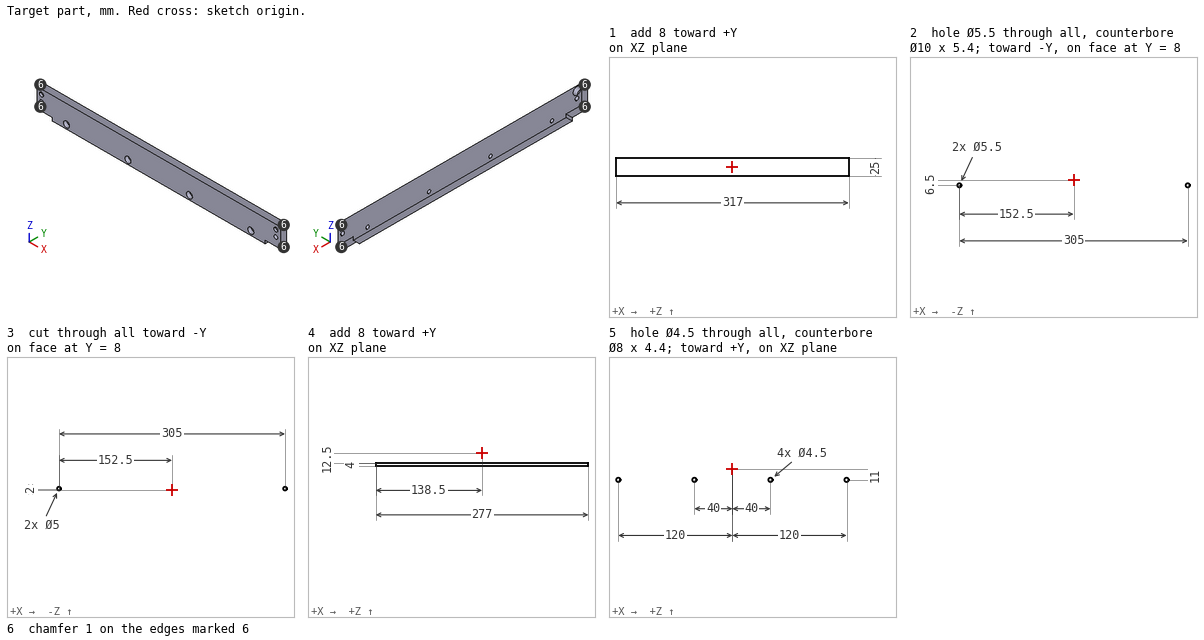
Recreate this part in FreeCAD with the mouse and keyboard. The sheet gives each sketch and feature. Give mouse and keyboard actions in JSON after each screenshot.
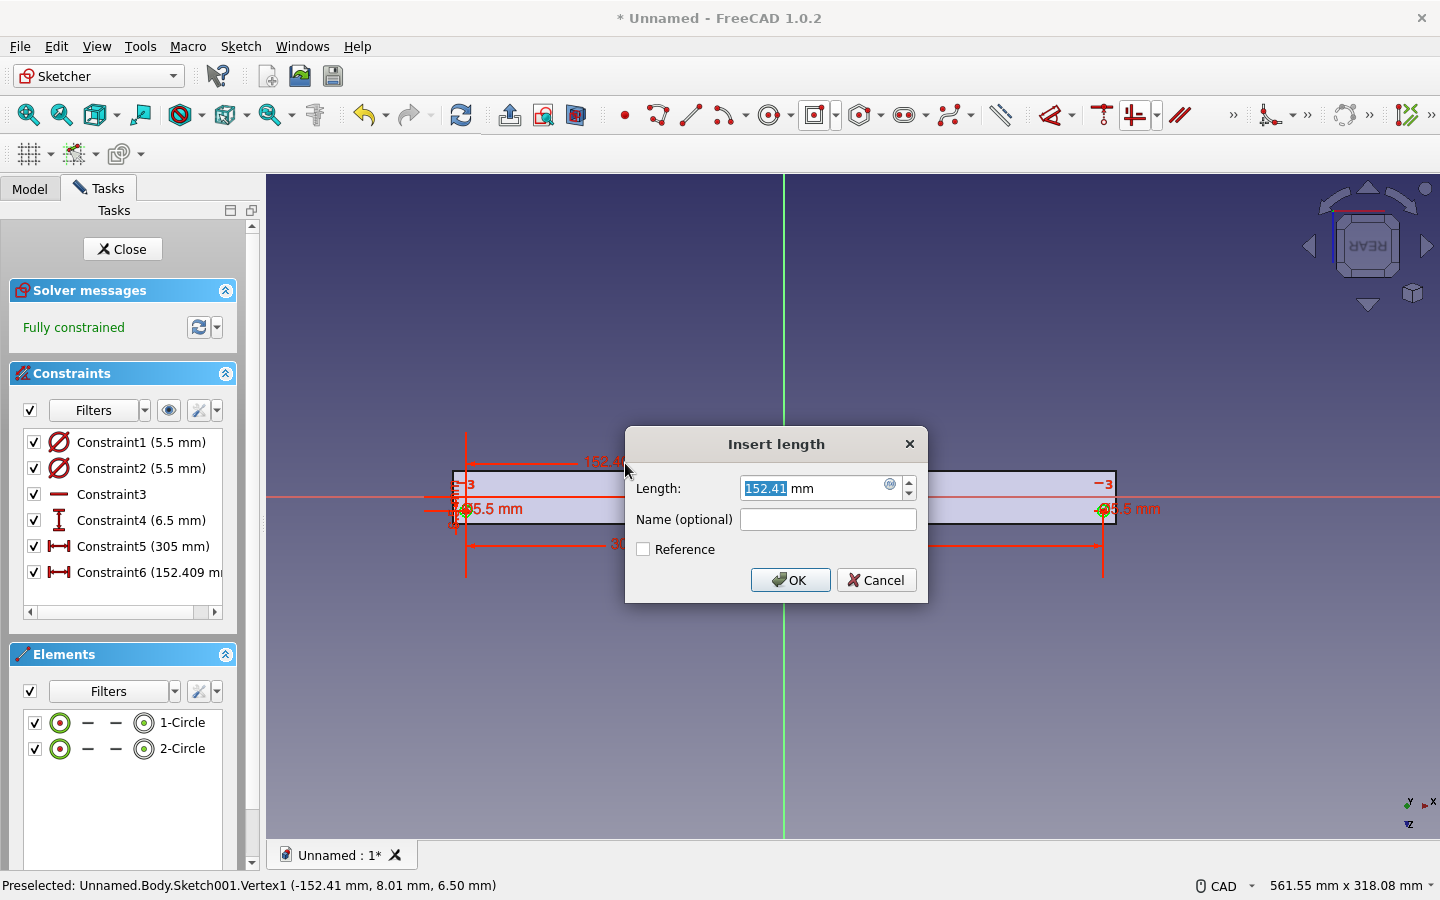
{"action": "type", "text": "152.5"}
{"action": "key", "text": "Return"}
{"action": "key", "text": "Escape"}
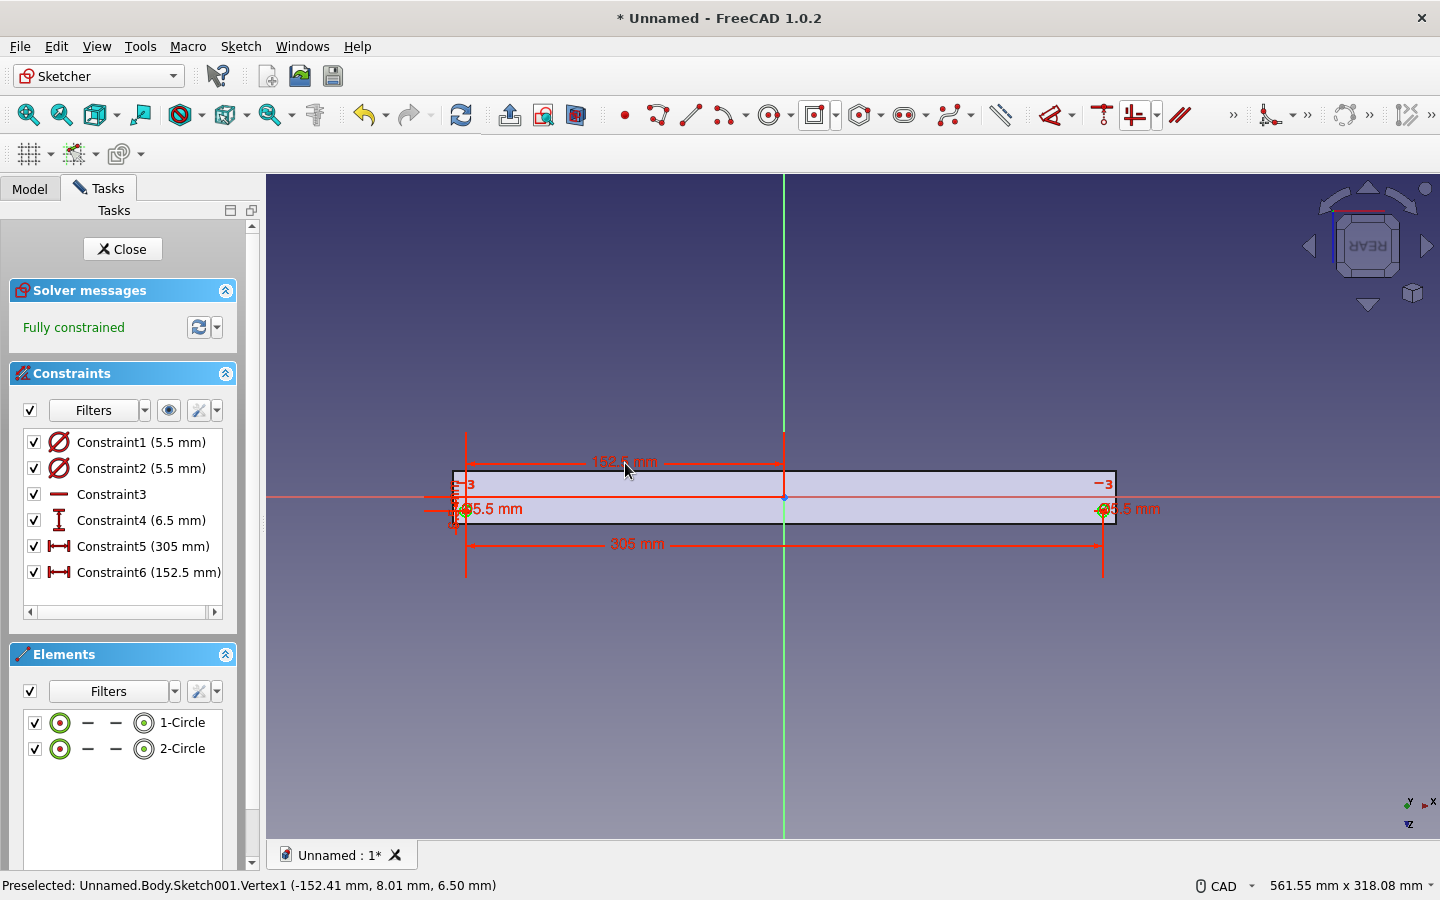
{"action": "left_click", "coordinate": [123, 249]}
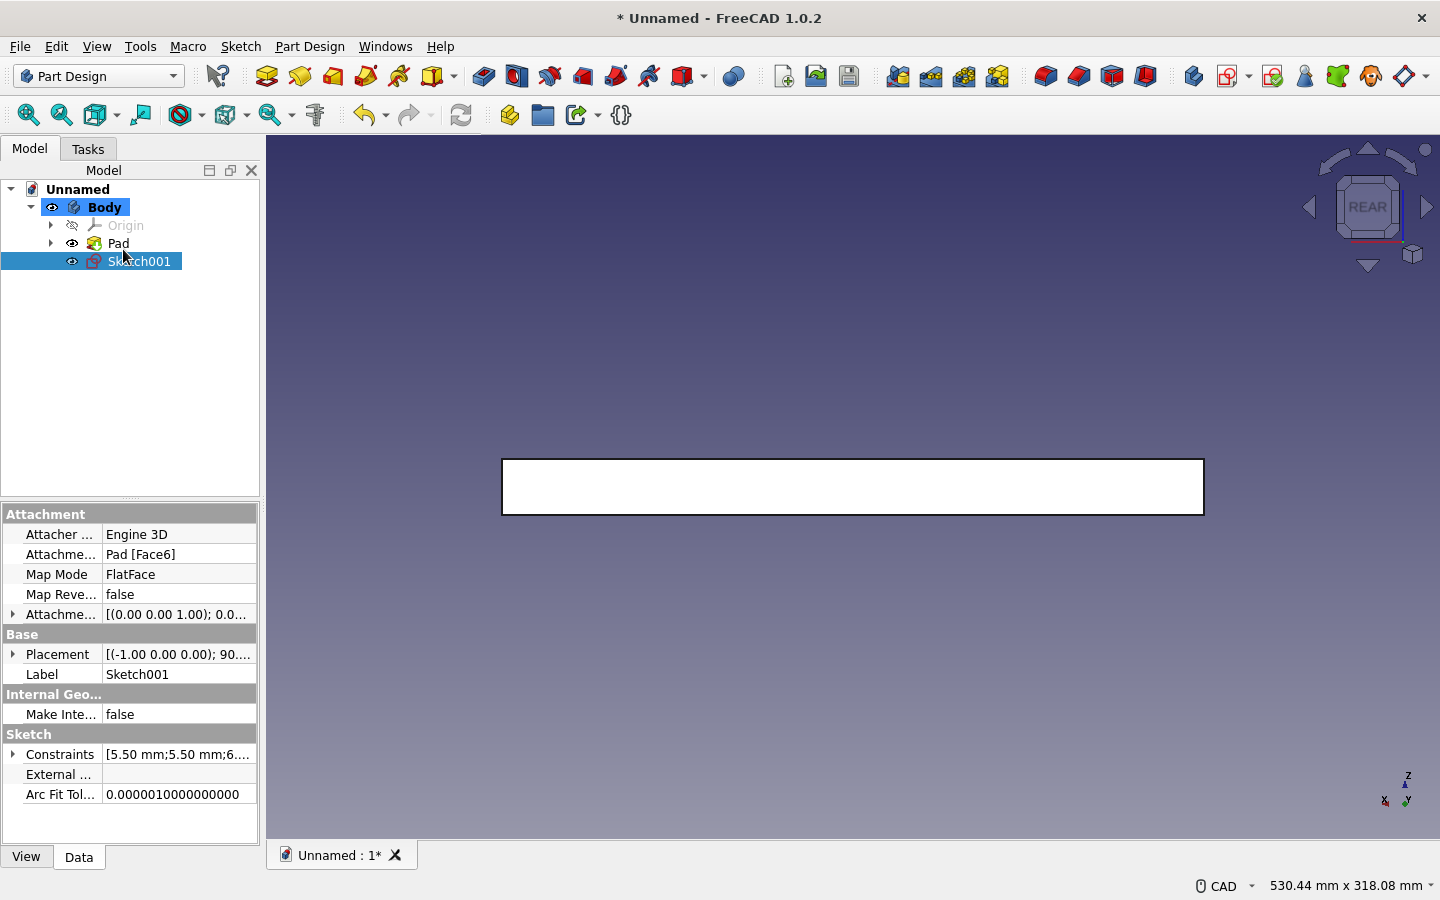
{"action": "left_click", "coordinate": [517, 76]}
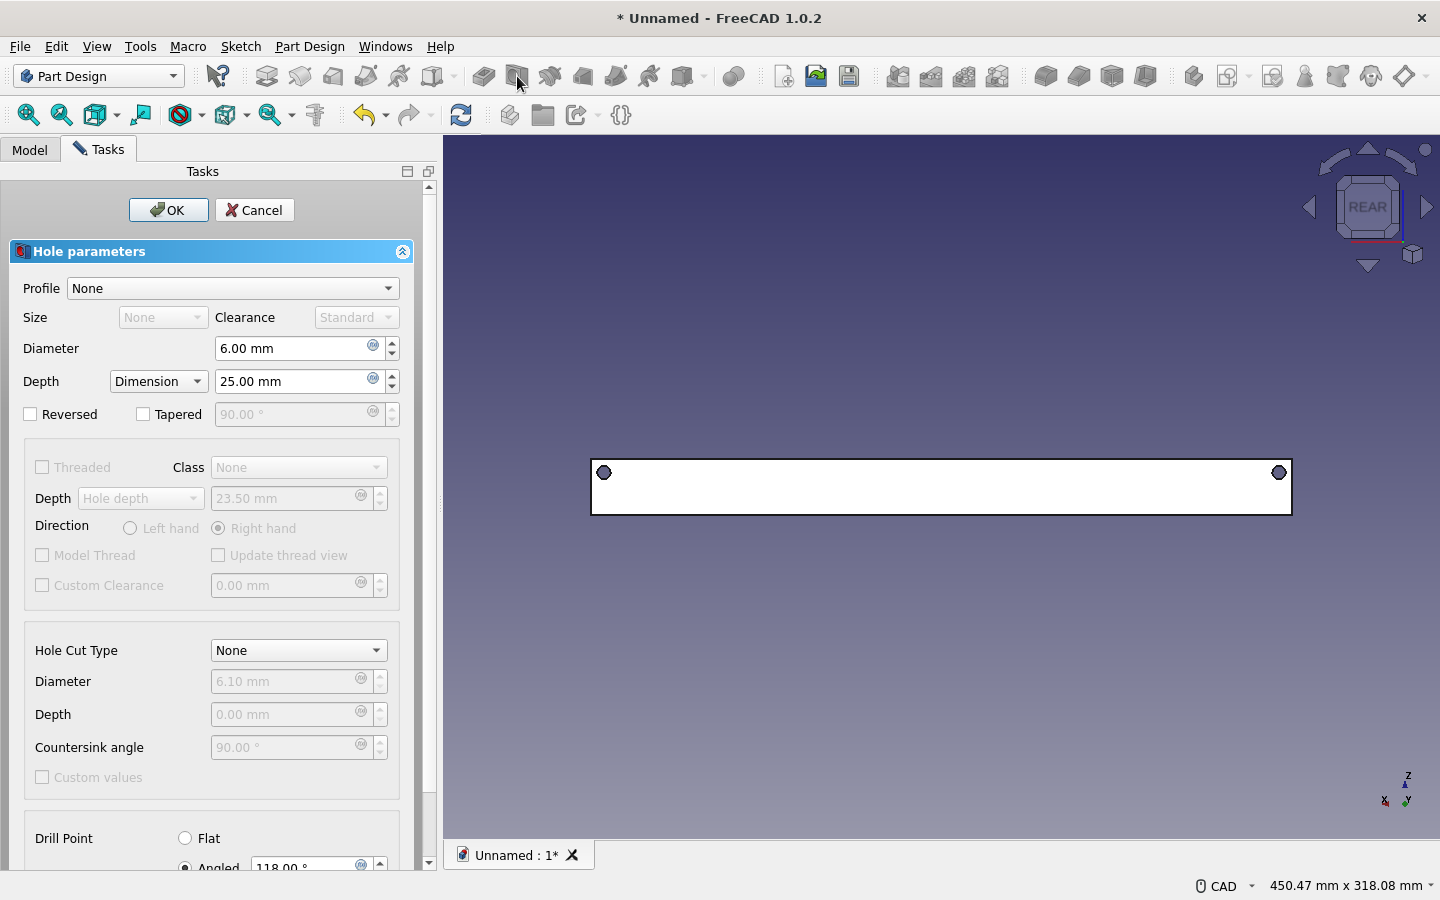
{"action": "triple_click", "coordinate": [300, 348]}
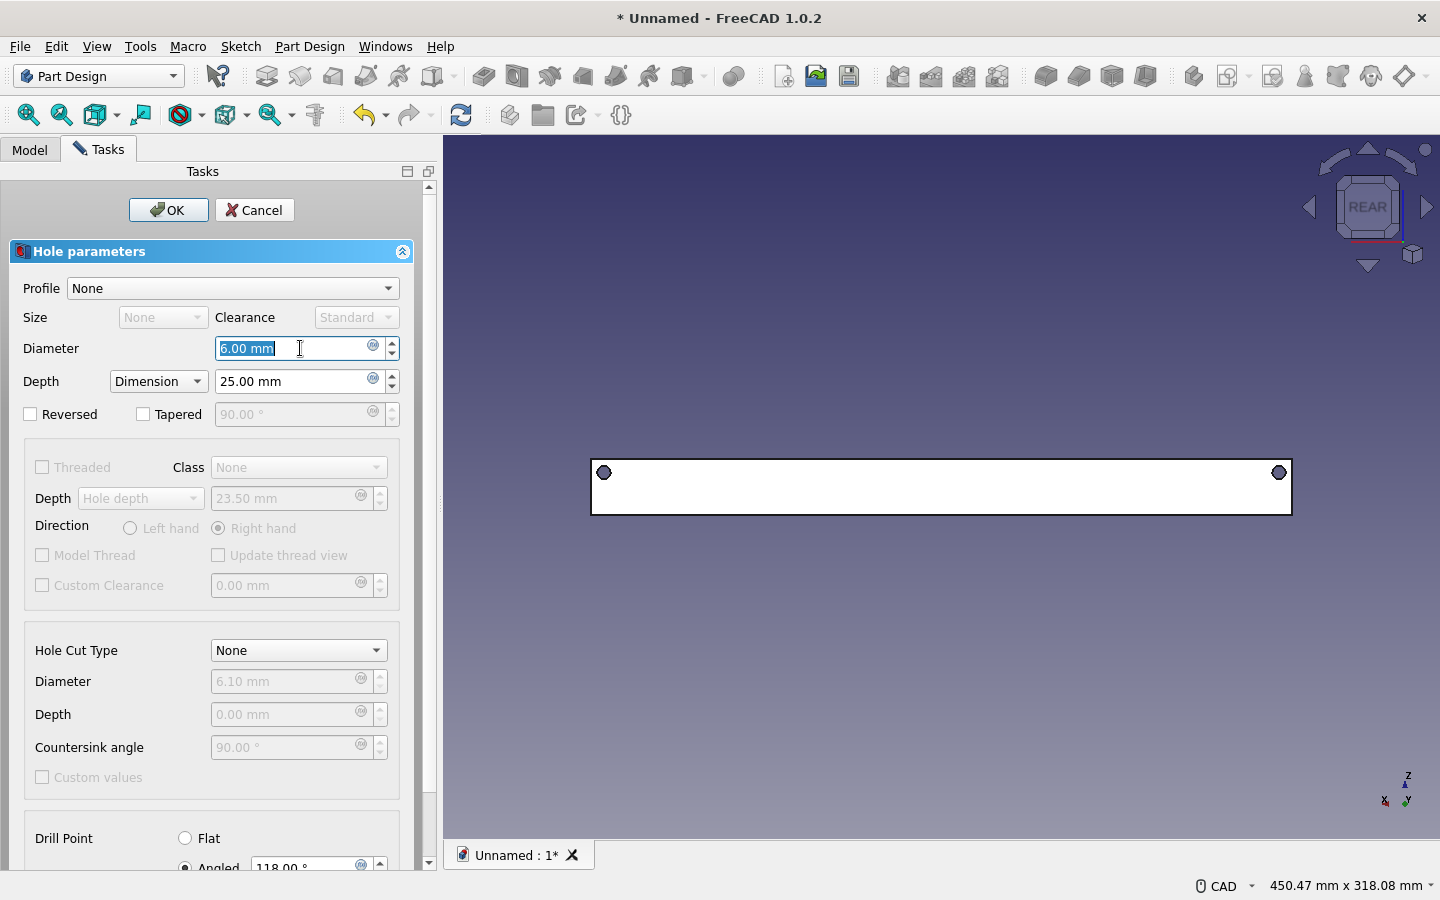
{"action": "type", "text": "5.5"}
{"action": "key", "text": "Tab"}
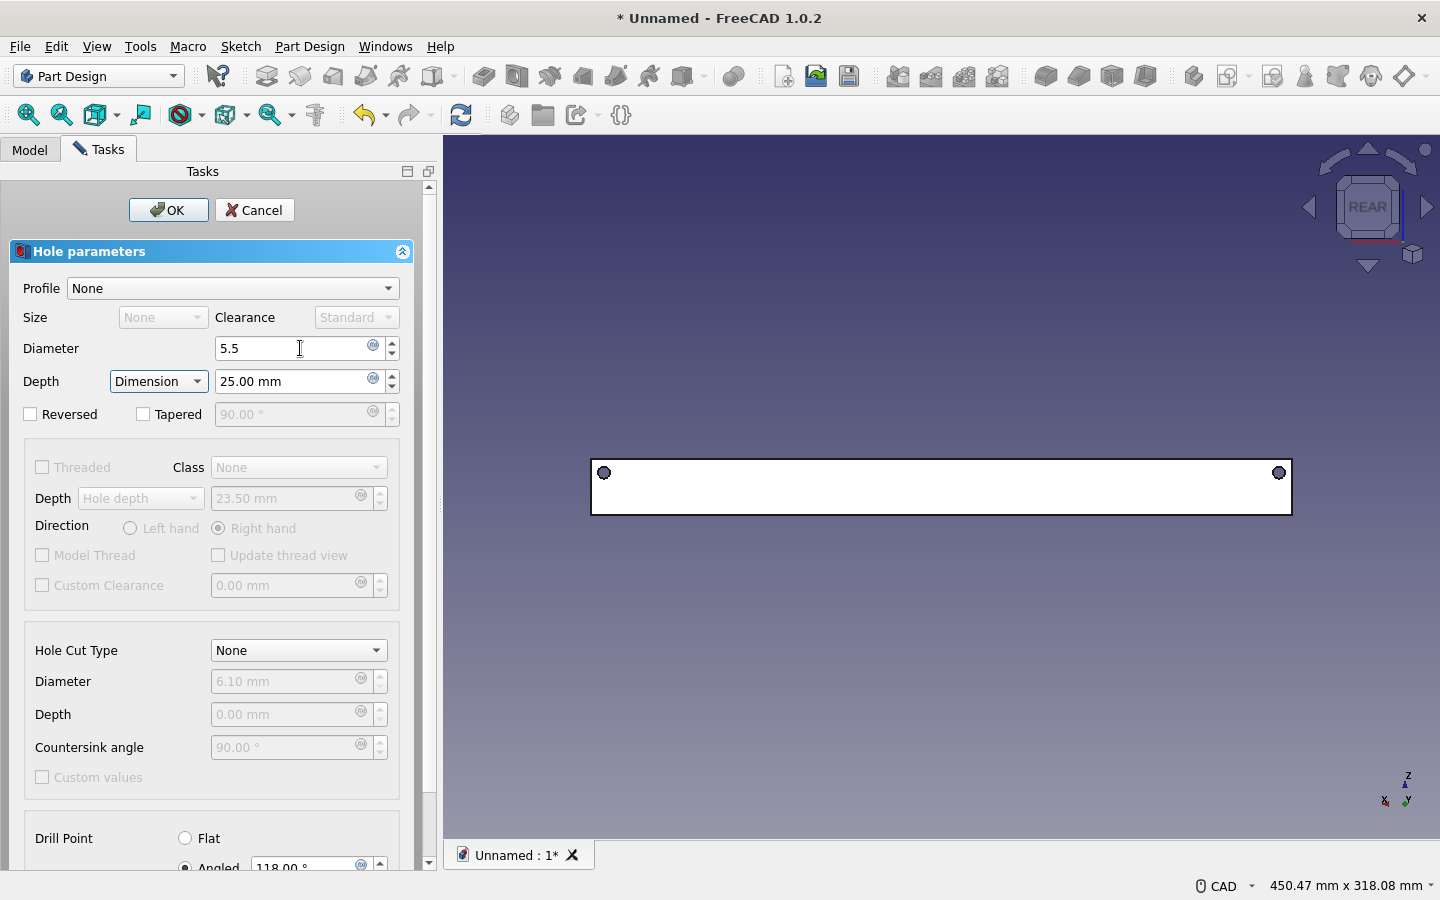
{"action": "left_click", "coordinate": [160, 382]}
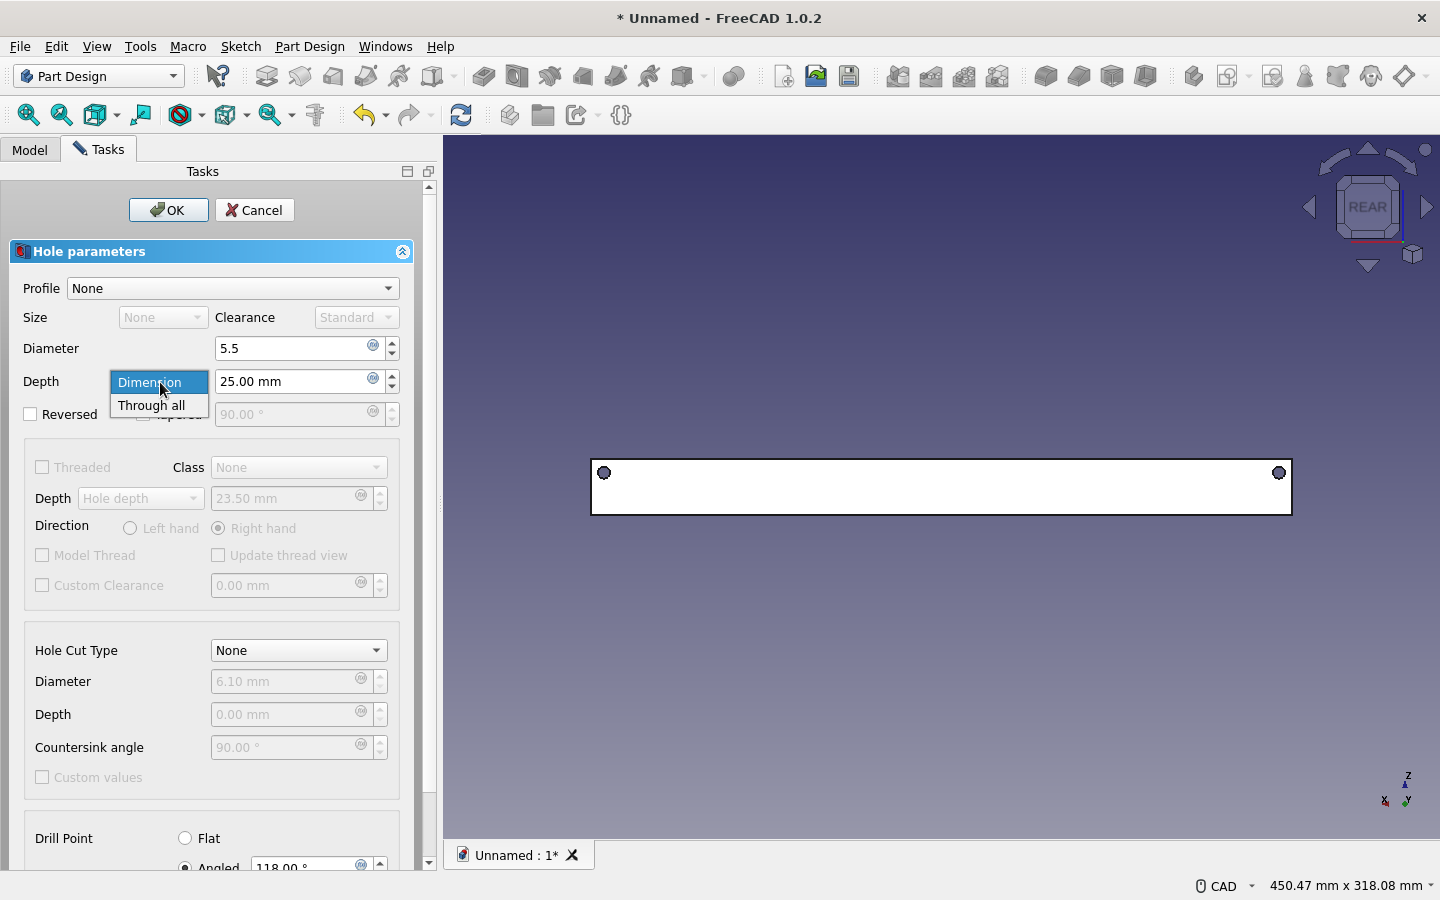
{"action": "left_click", "coordinate": [158, 406]}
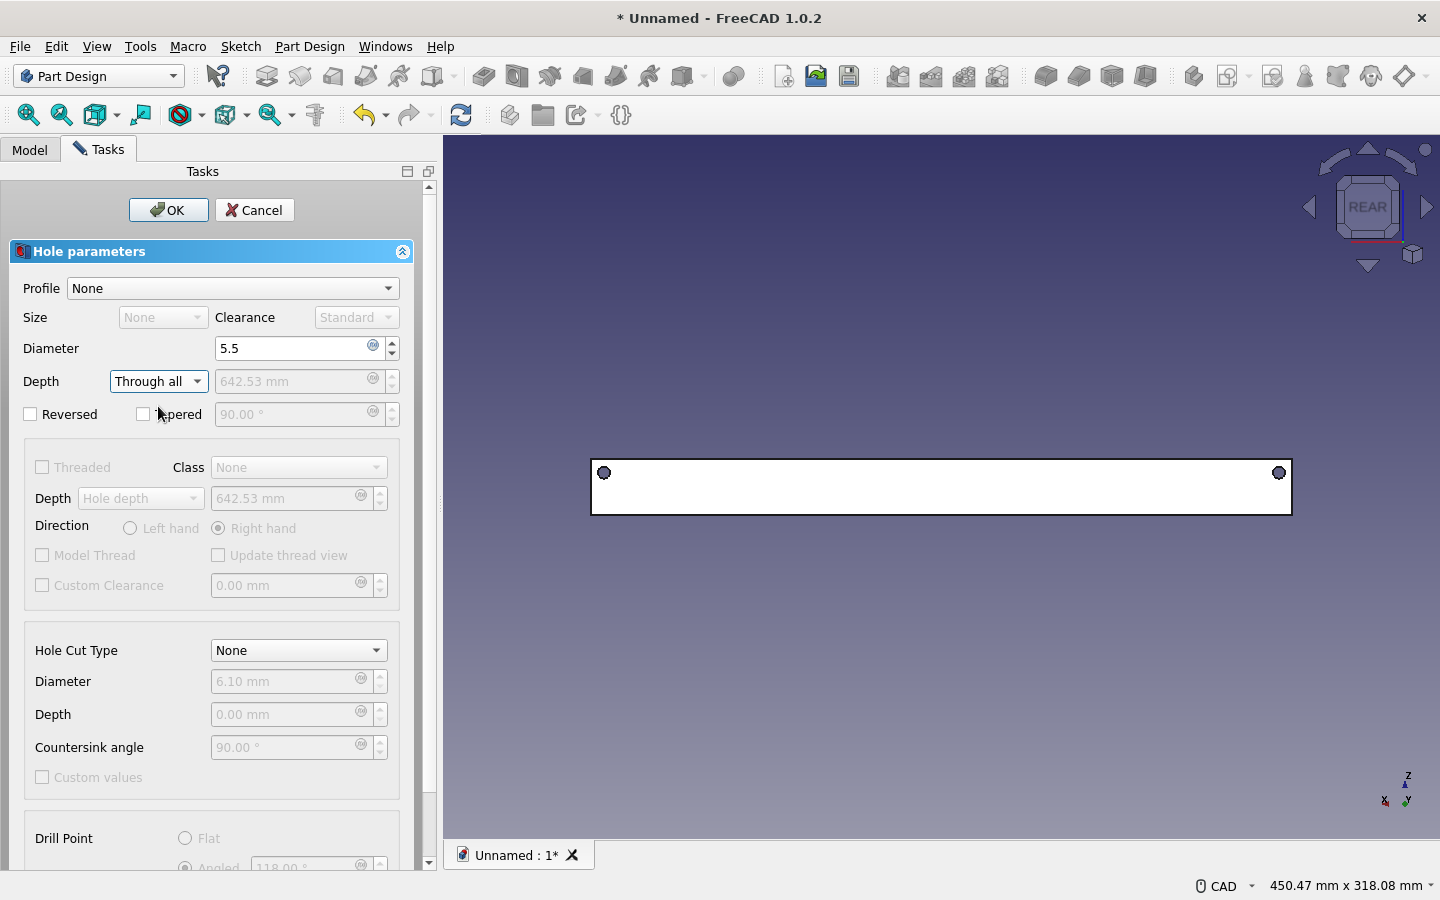
{"action": "left_click", "coordinate": [300, 650]}